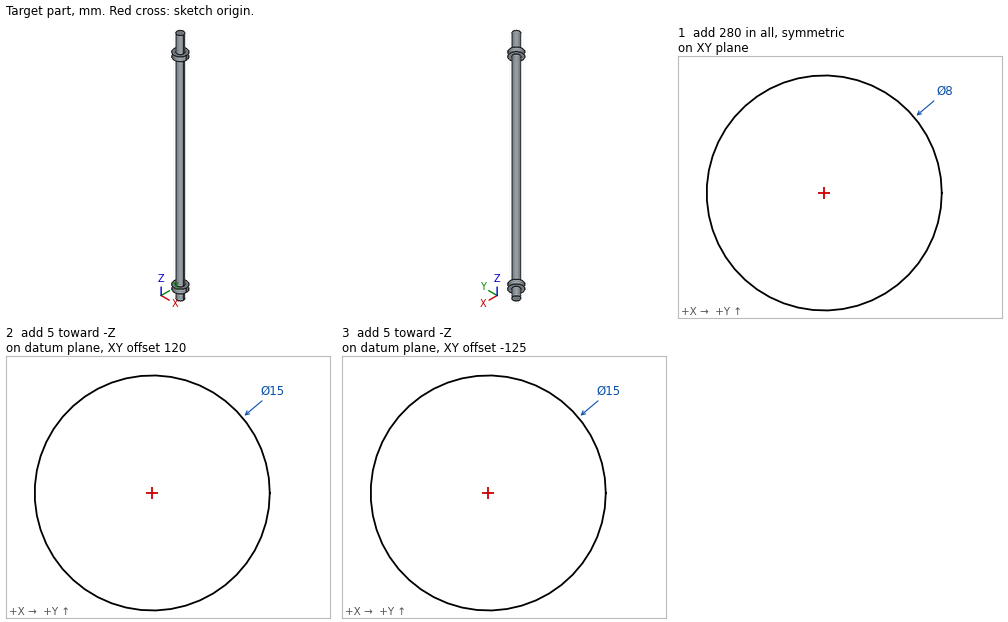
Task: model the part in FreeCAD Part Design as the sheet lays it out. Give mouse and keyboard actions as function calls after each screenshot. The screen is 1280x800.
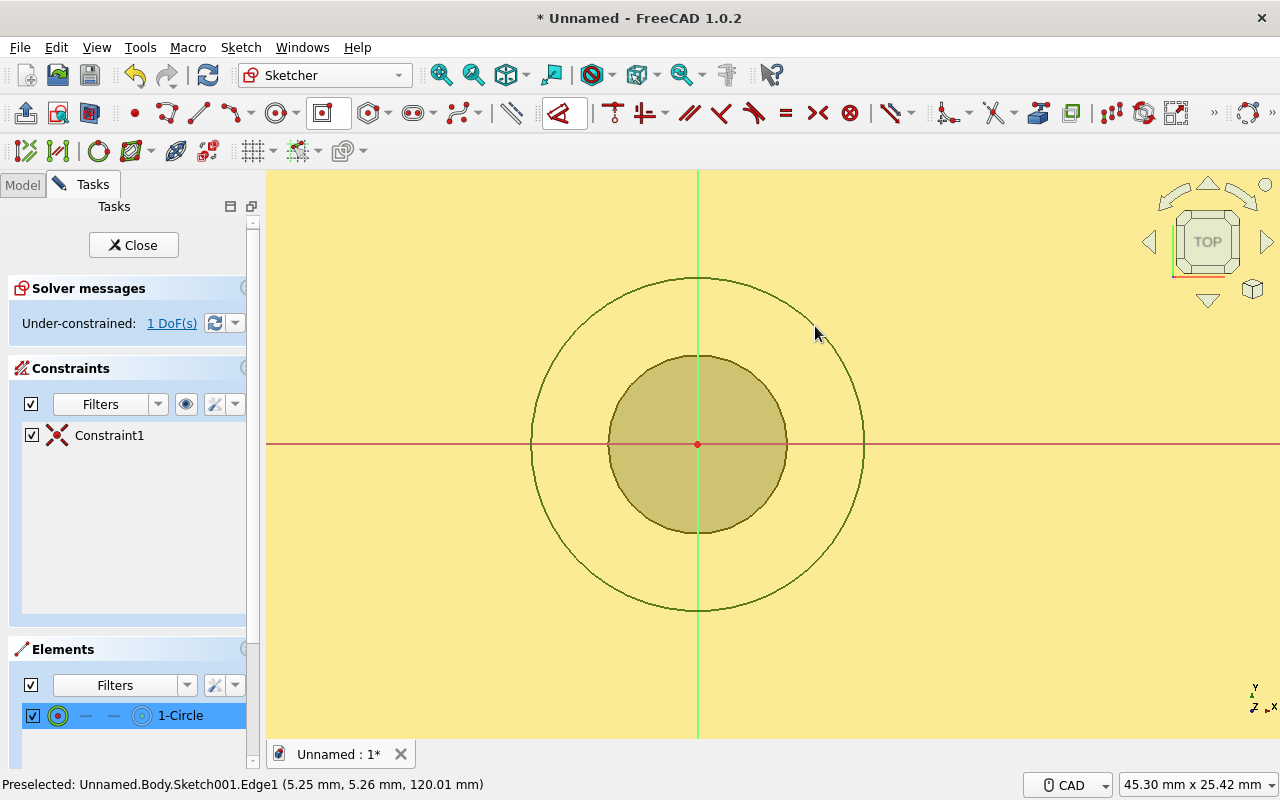
key(k)
key(o)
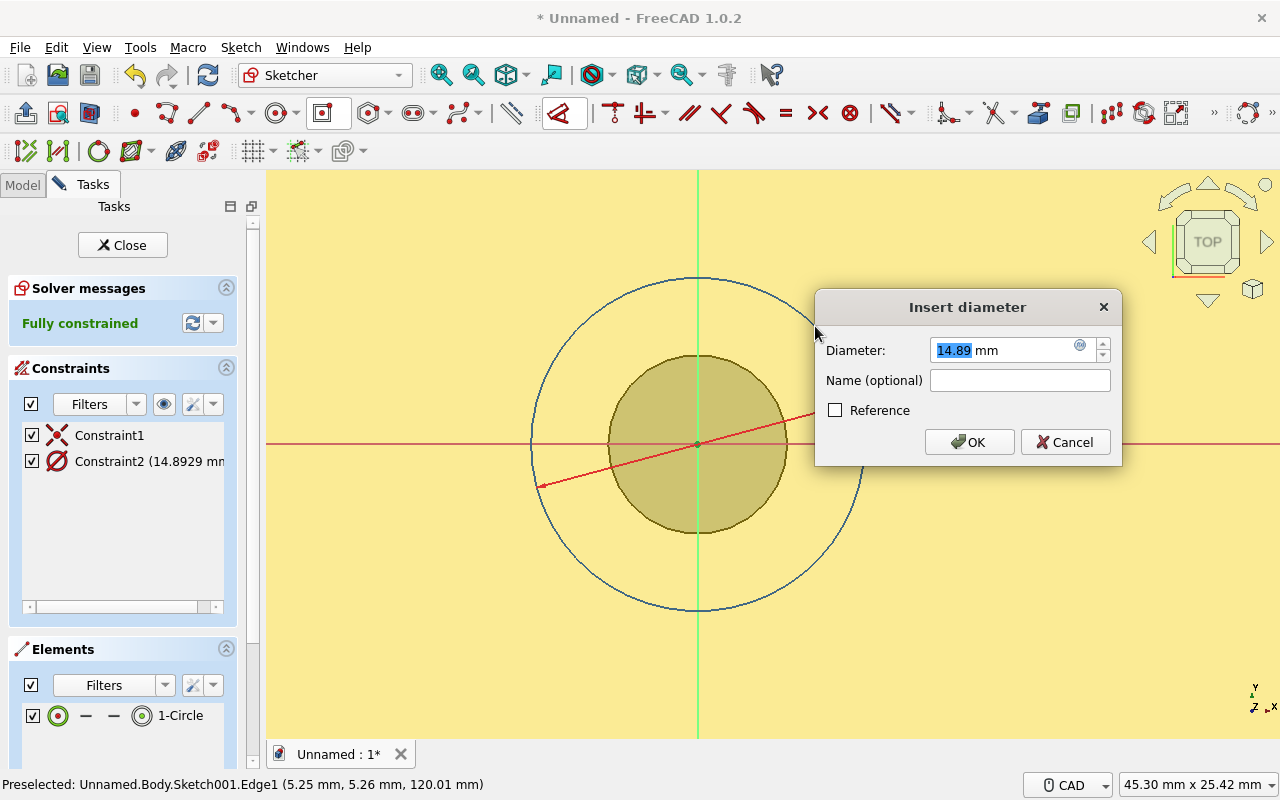
text(15)
key(Return)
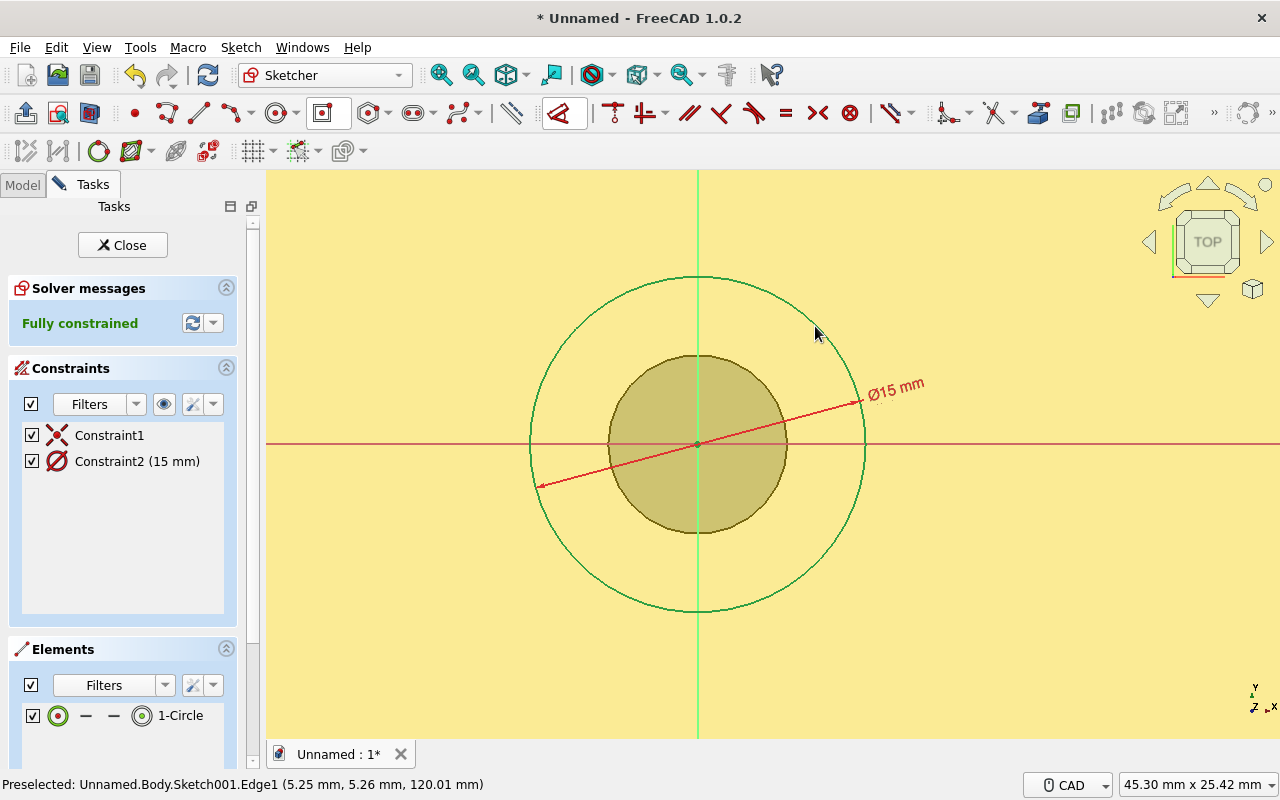
click(123, 245)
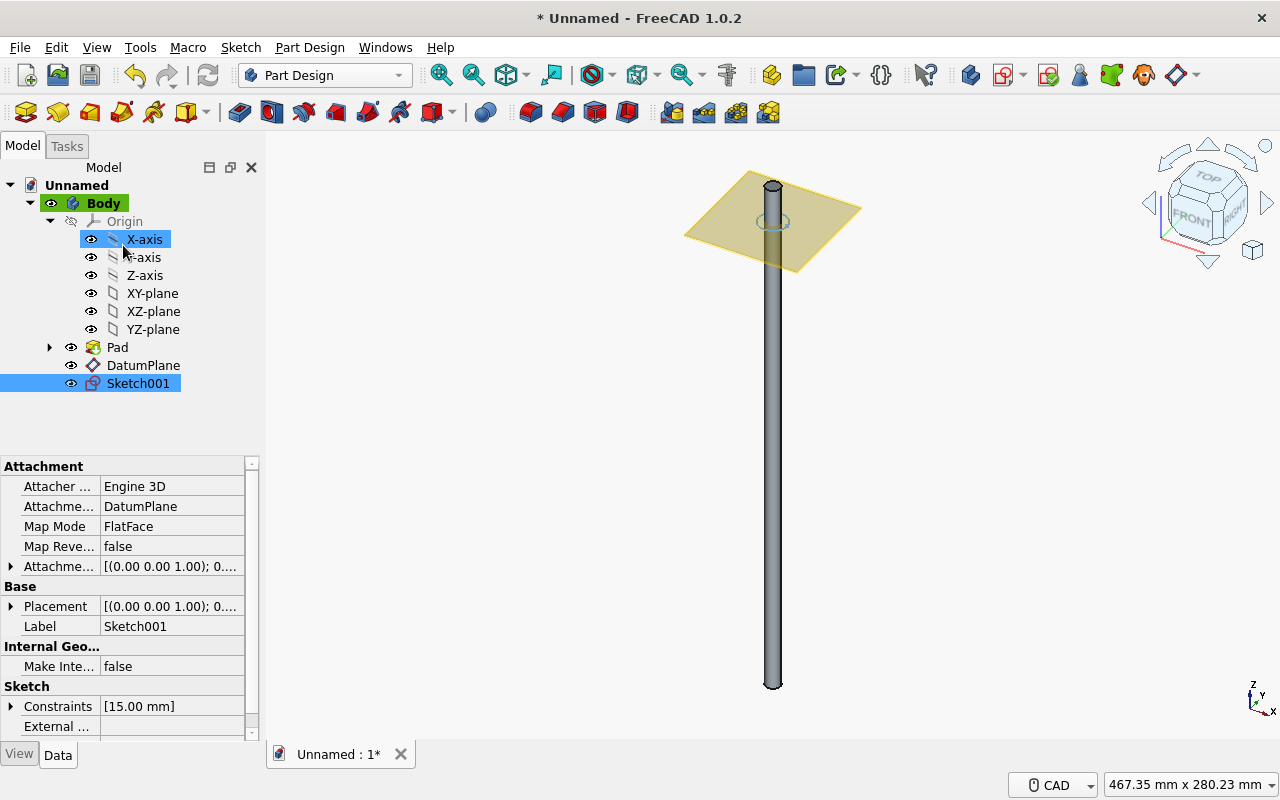
click(26, 112)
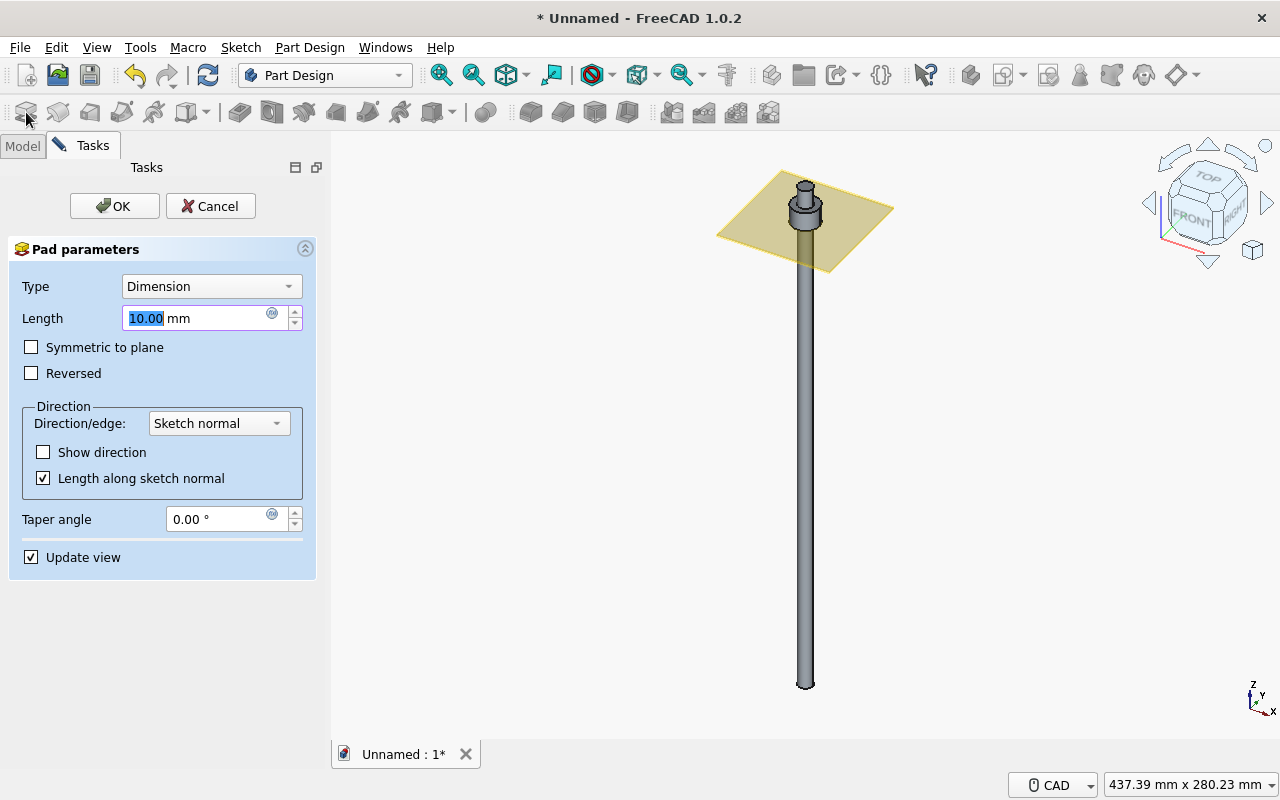
text(5)
key(Tab)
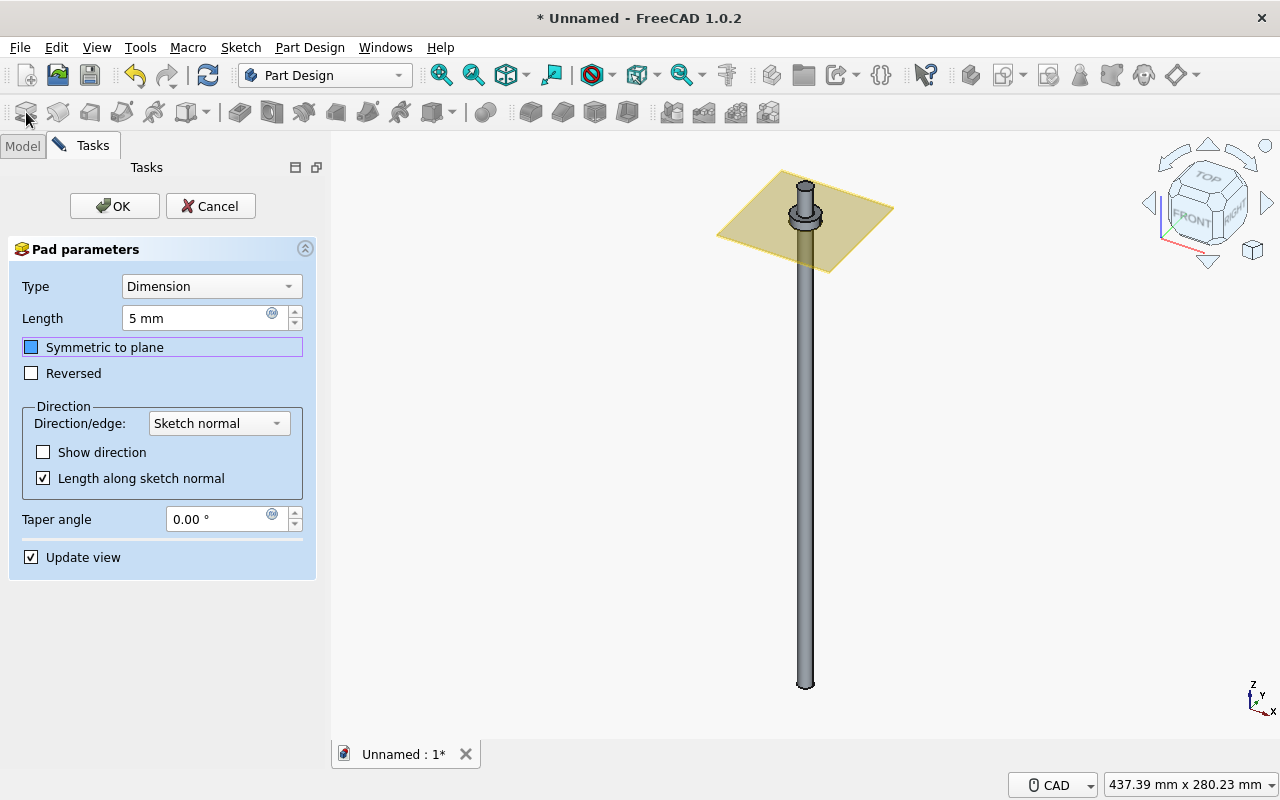
click(30, 373)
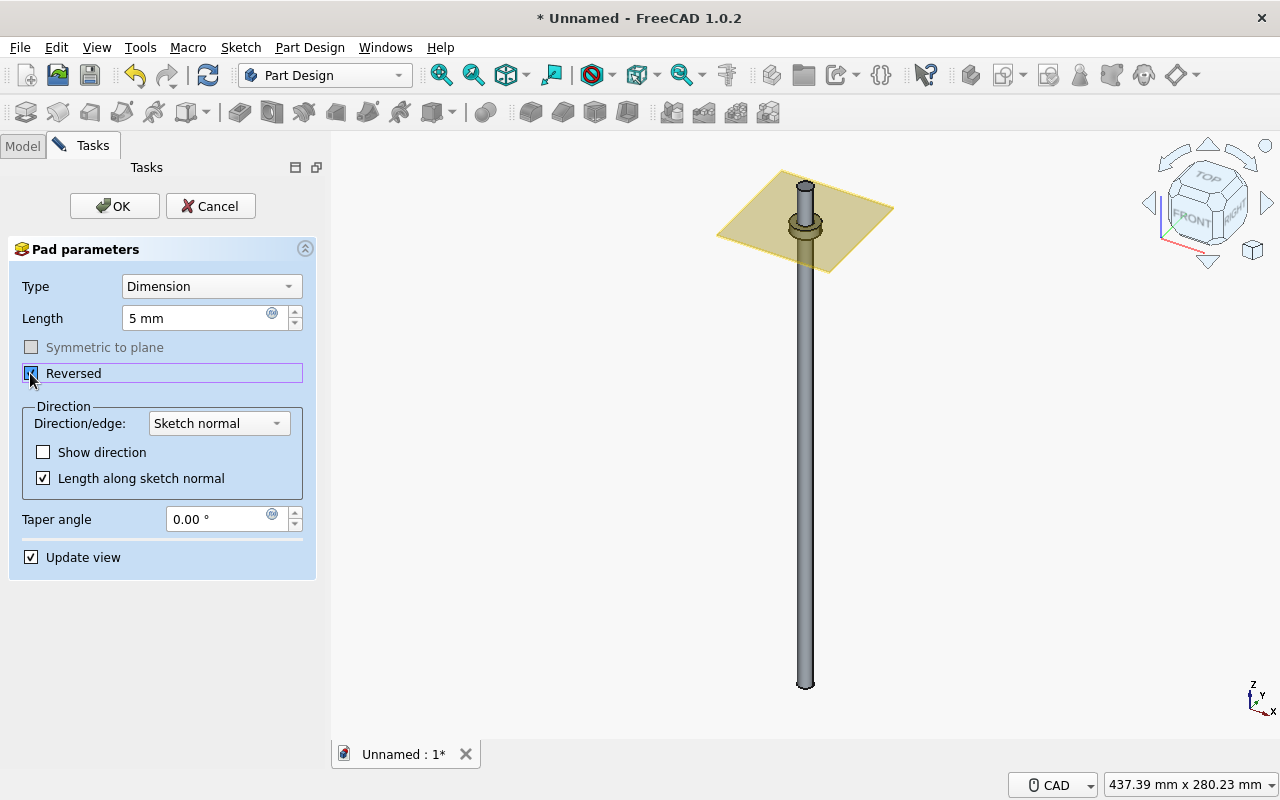
click(115, 206)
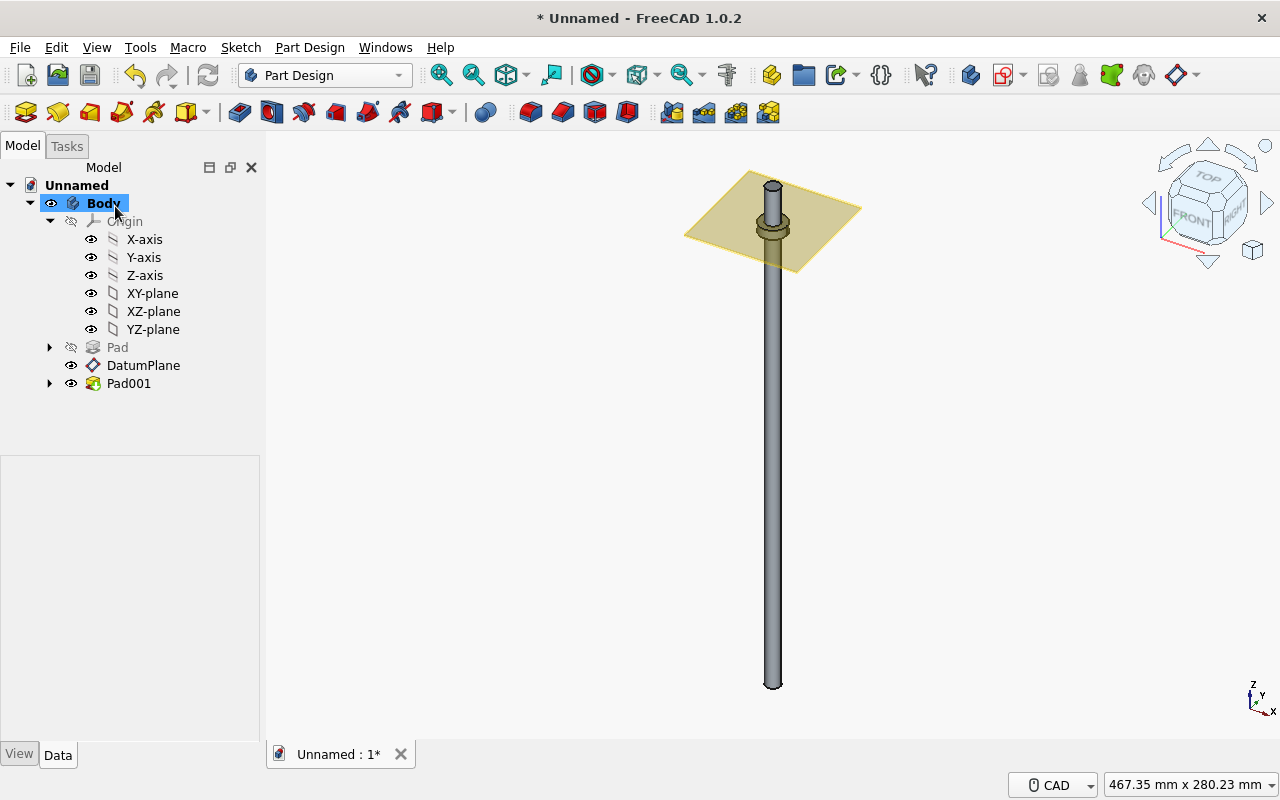
click(116, 365)
key(space)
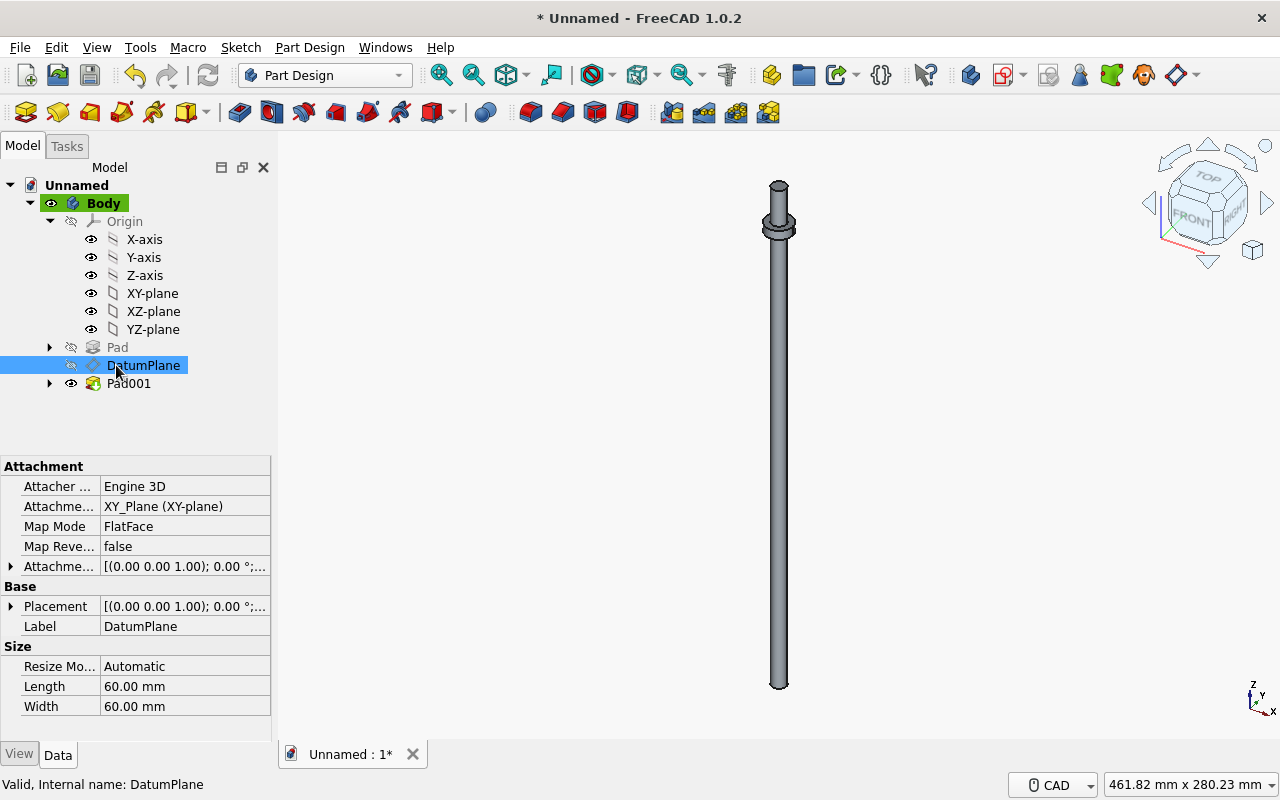
click(136, 293)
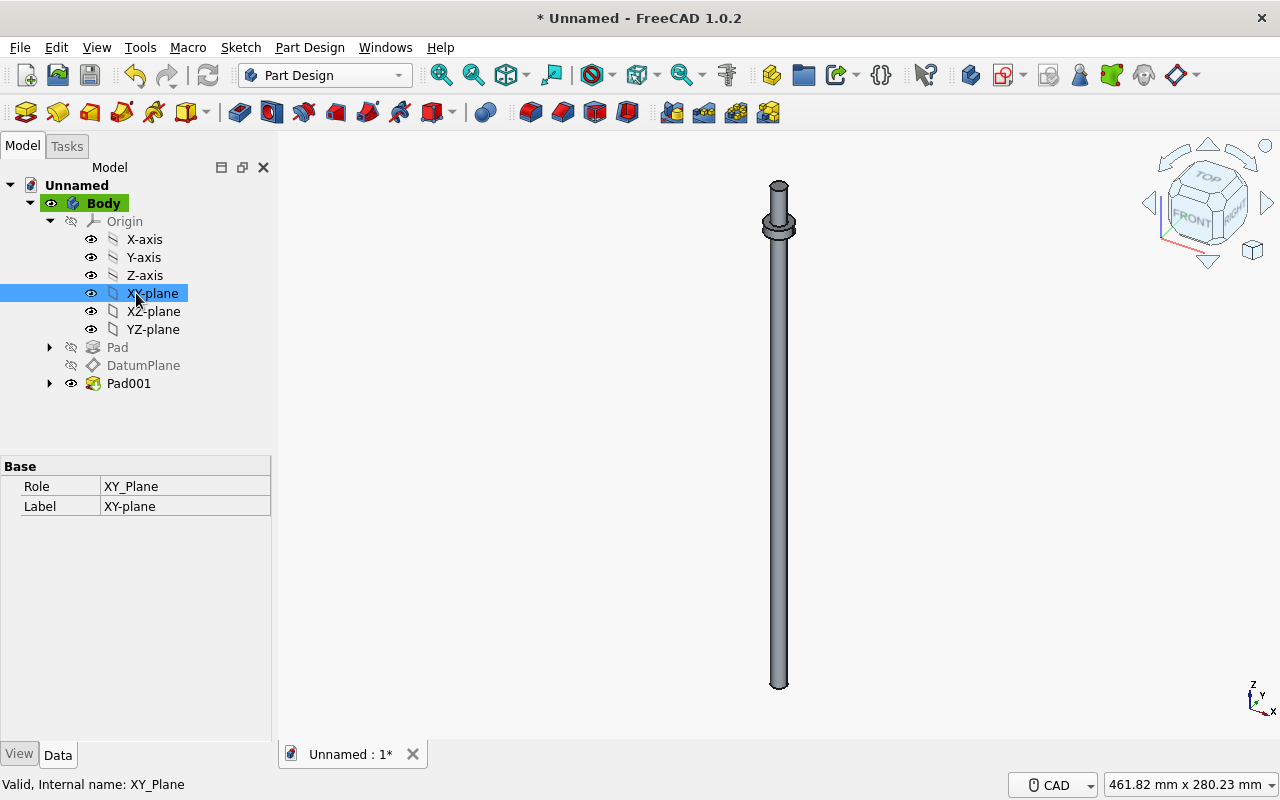
click(1176, 76)